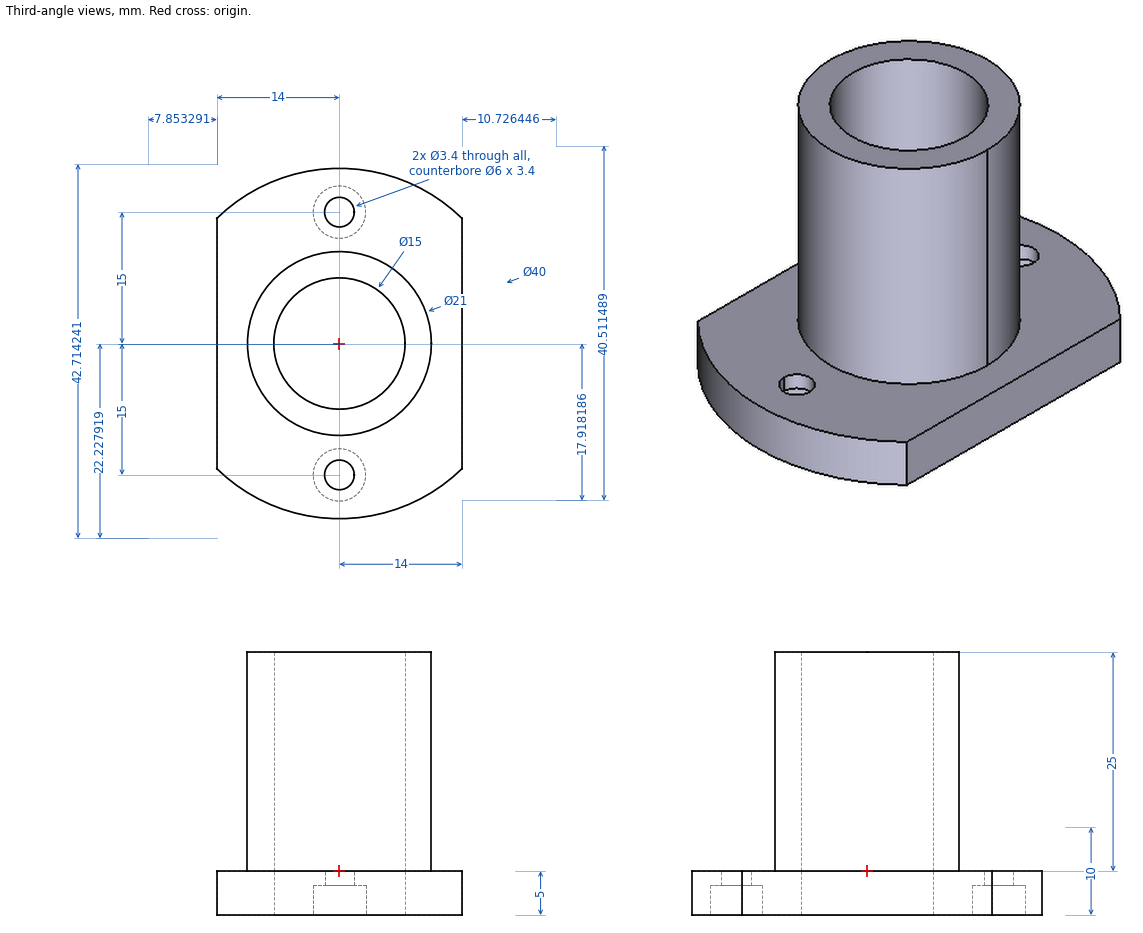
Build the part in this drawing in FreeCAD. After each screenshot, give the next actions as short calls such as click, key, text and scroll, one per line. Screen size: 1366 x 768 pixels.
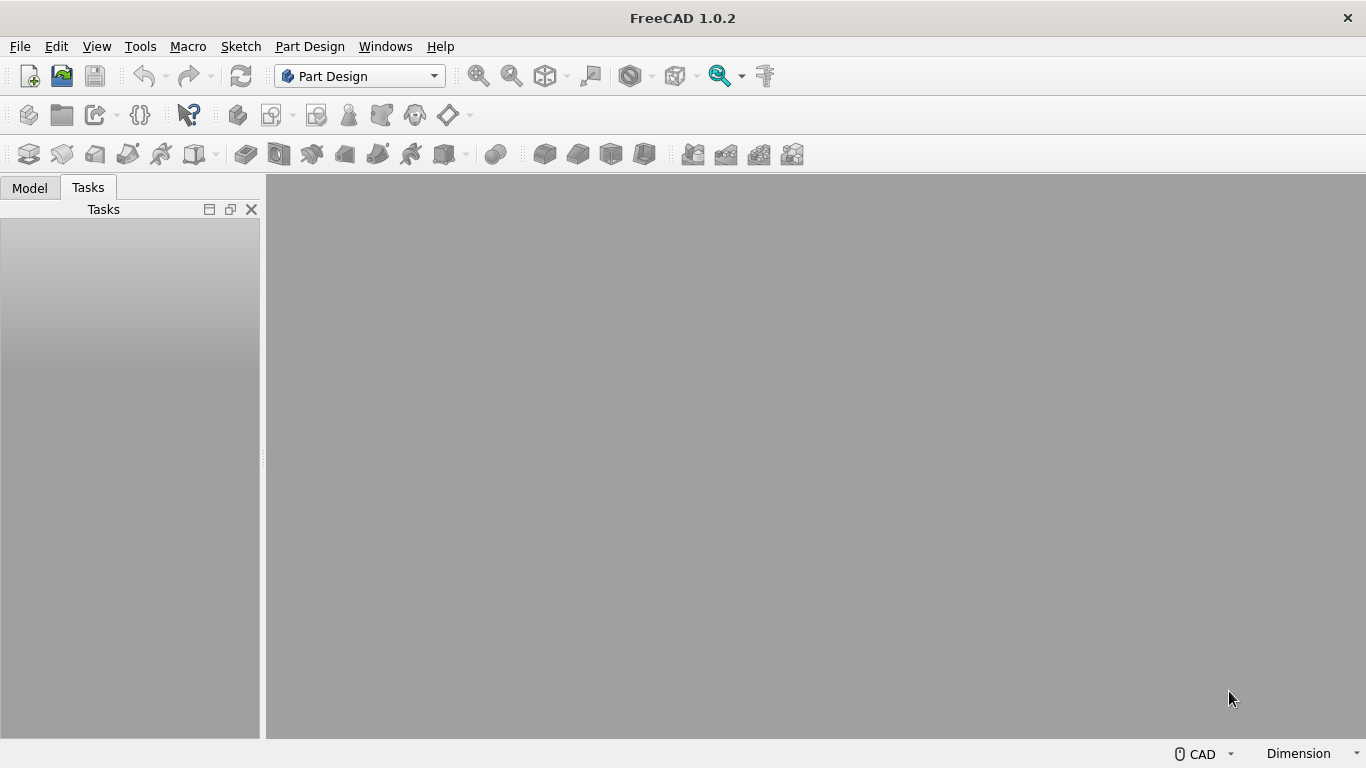
click(29, 76)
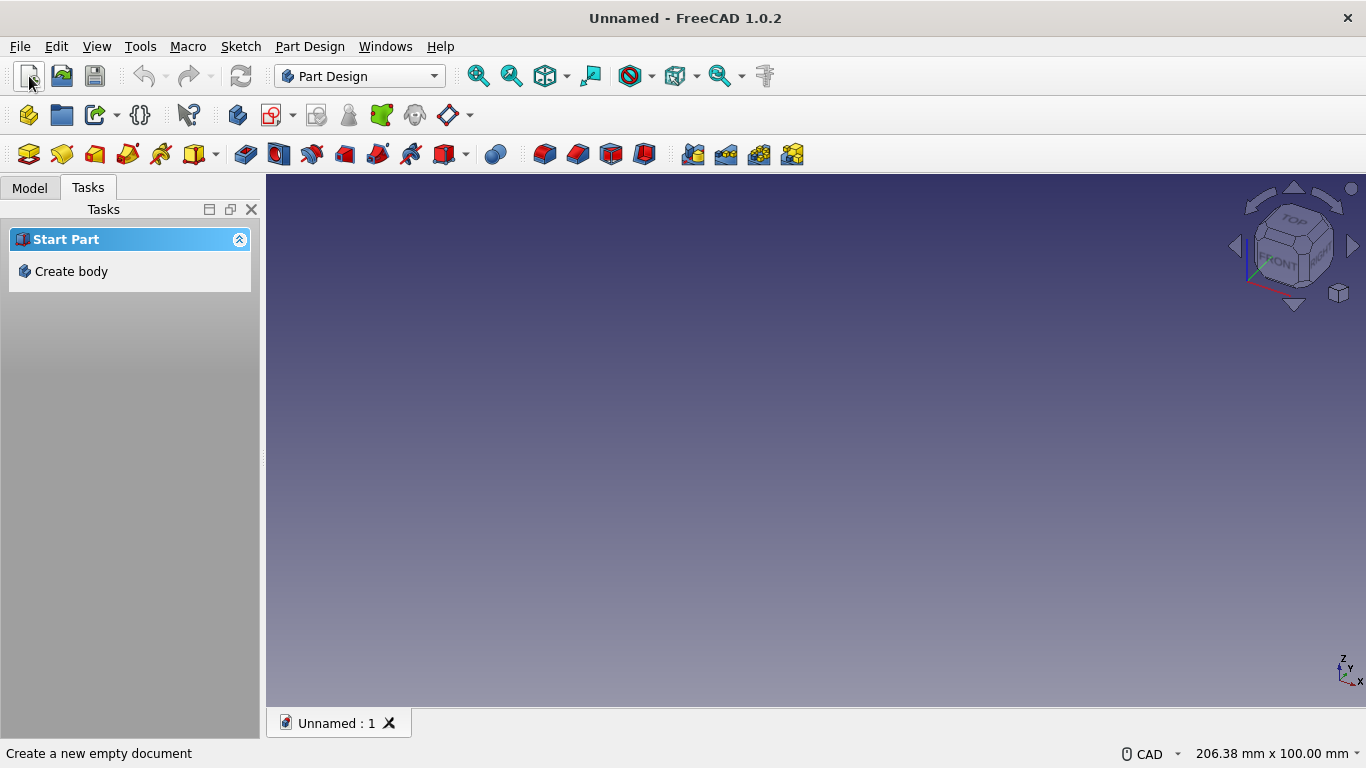
click(270, 116)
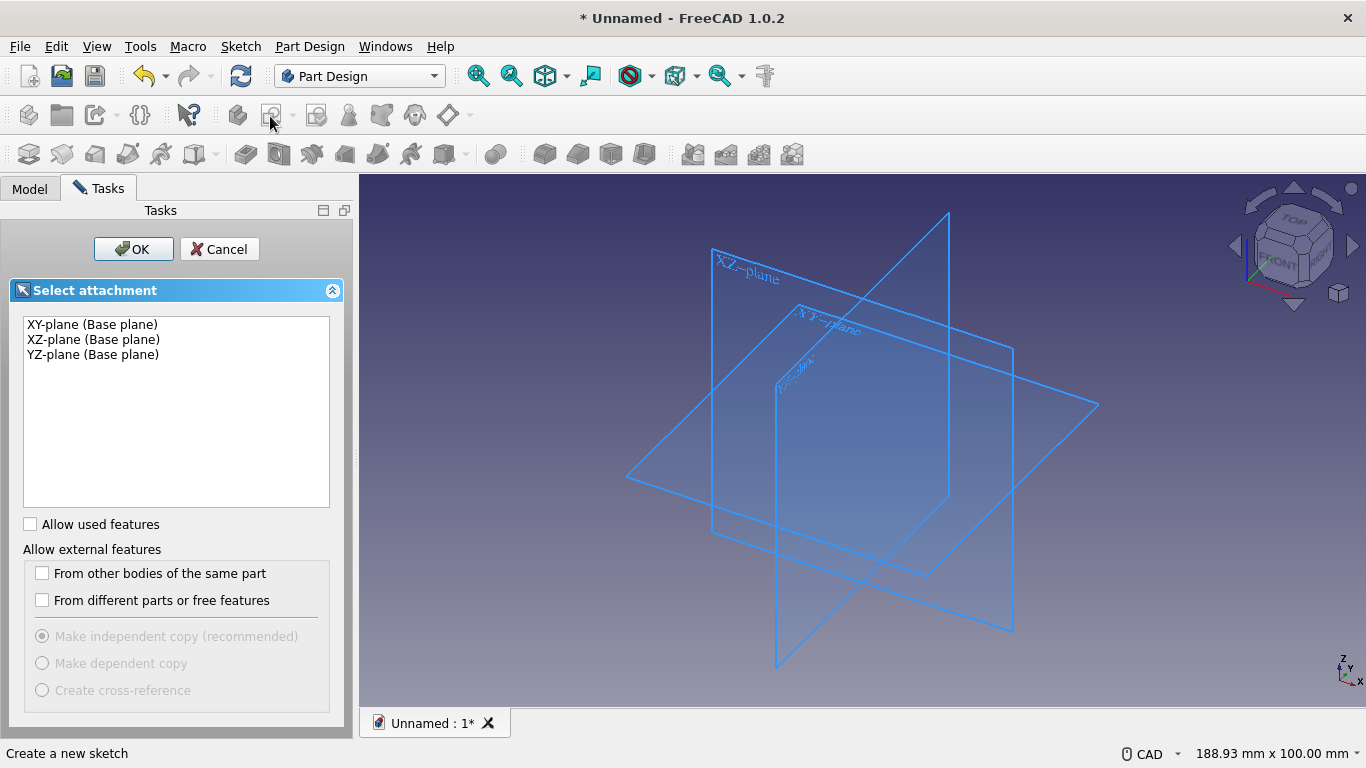
click(84, 324)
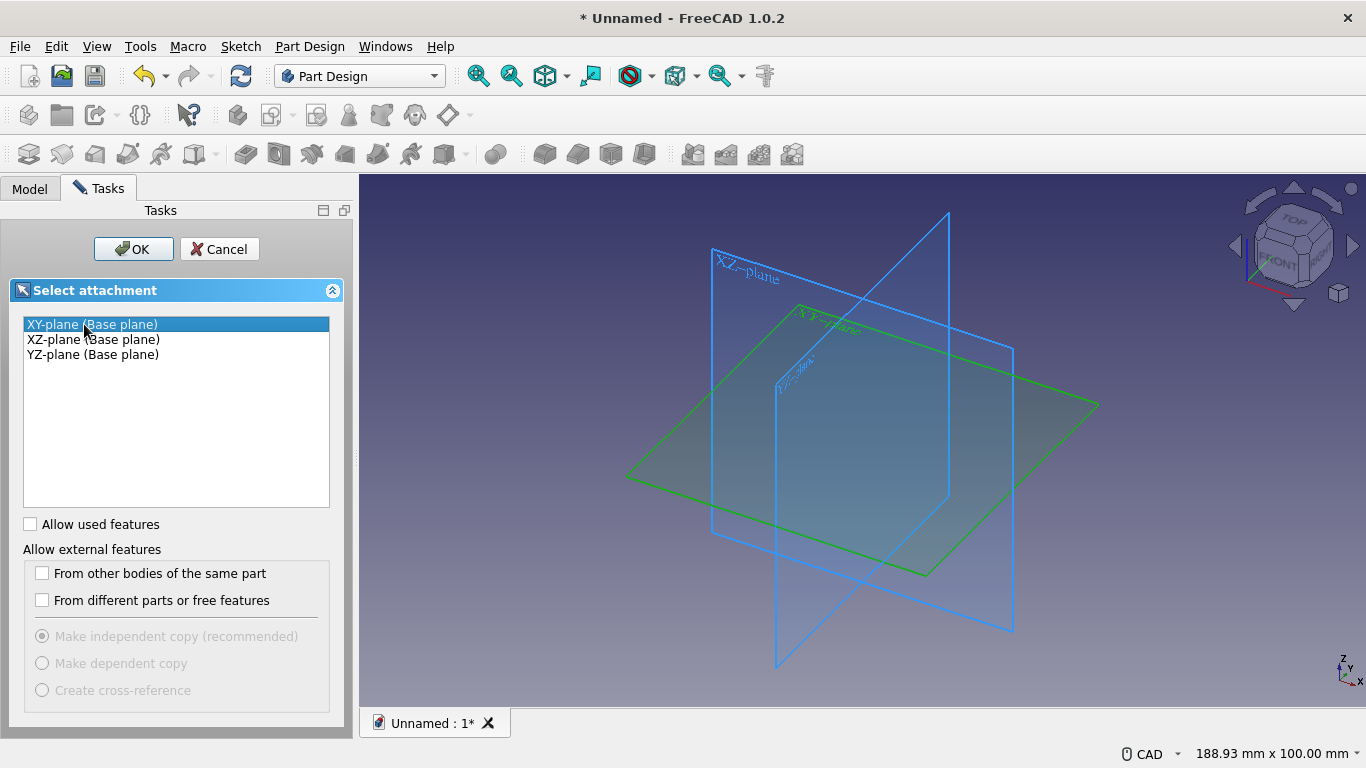
click(134, 249)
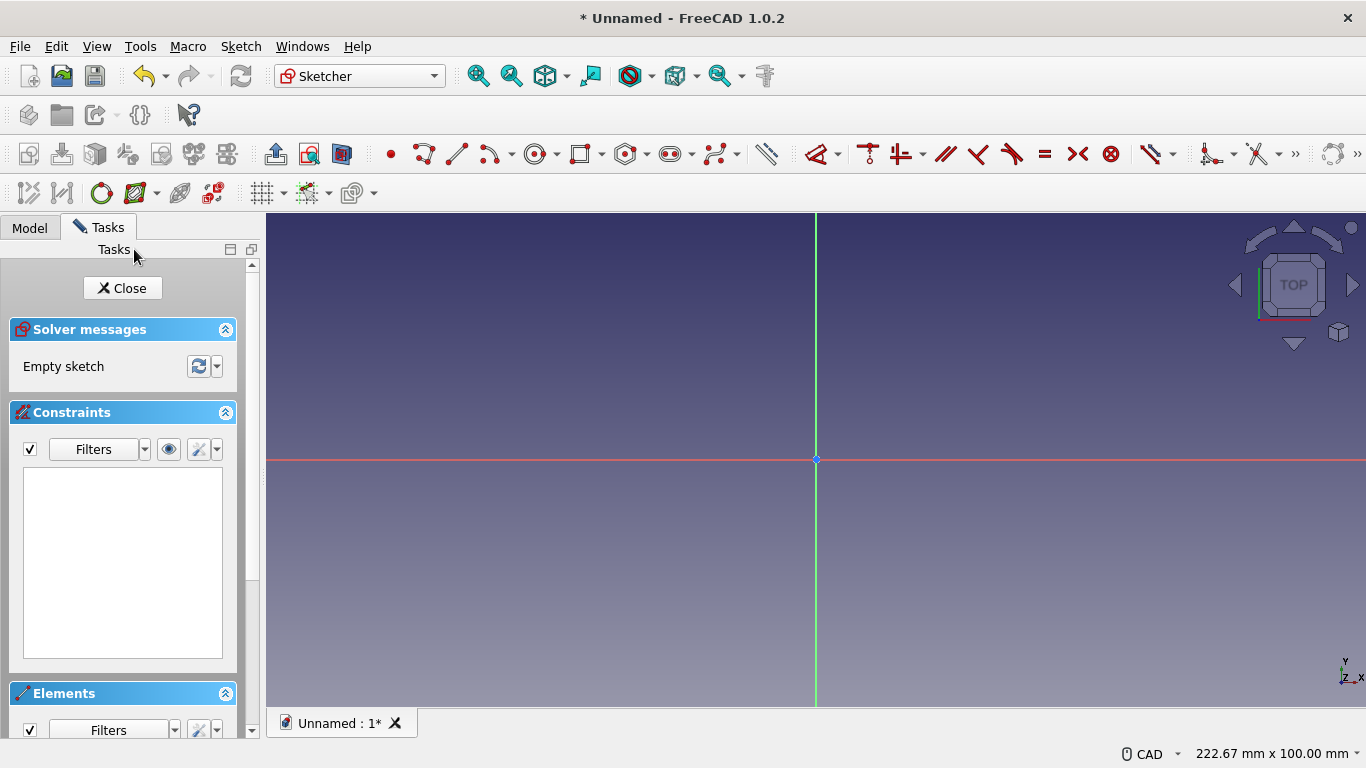
scroll(856, 460, up, 5)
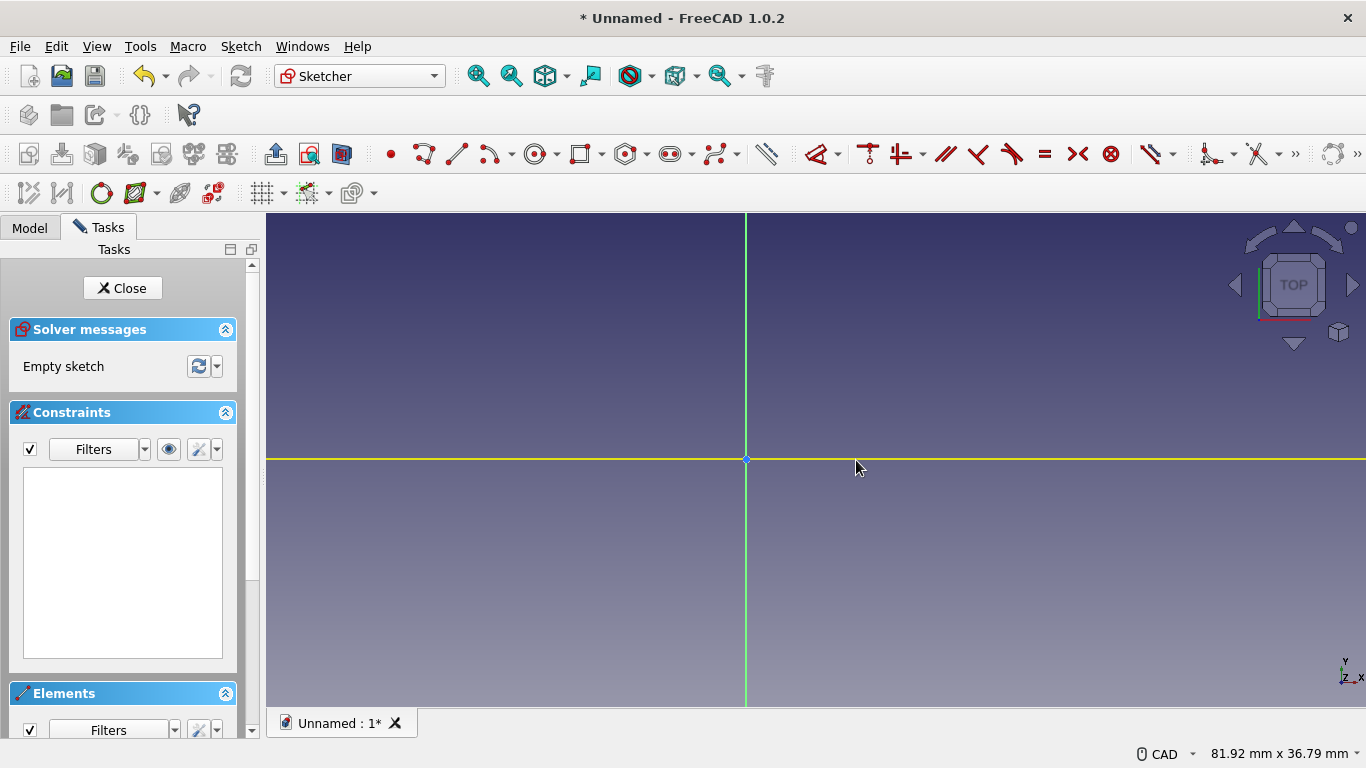
click(534, 154)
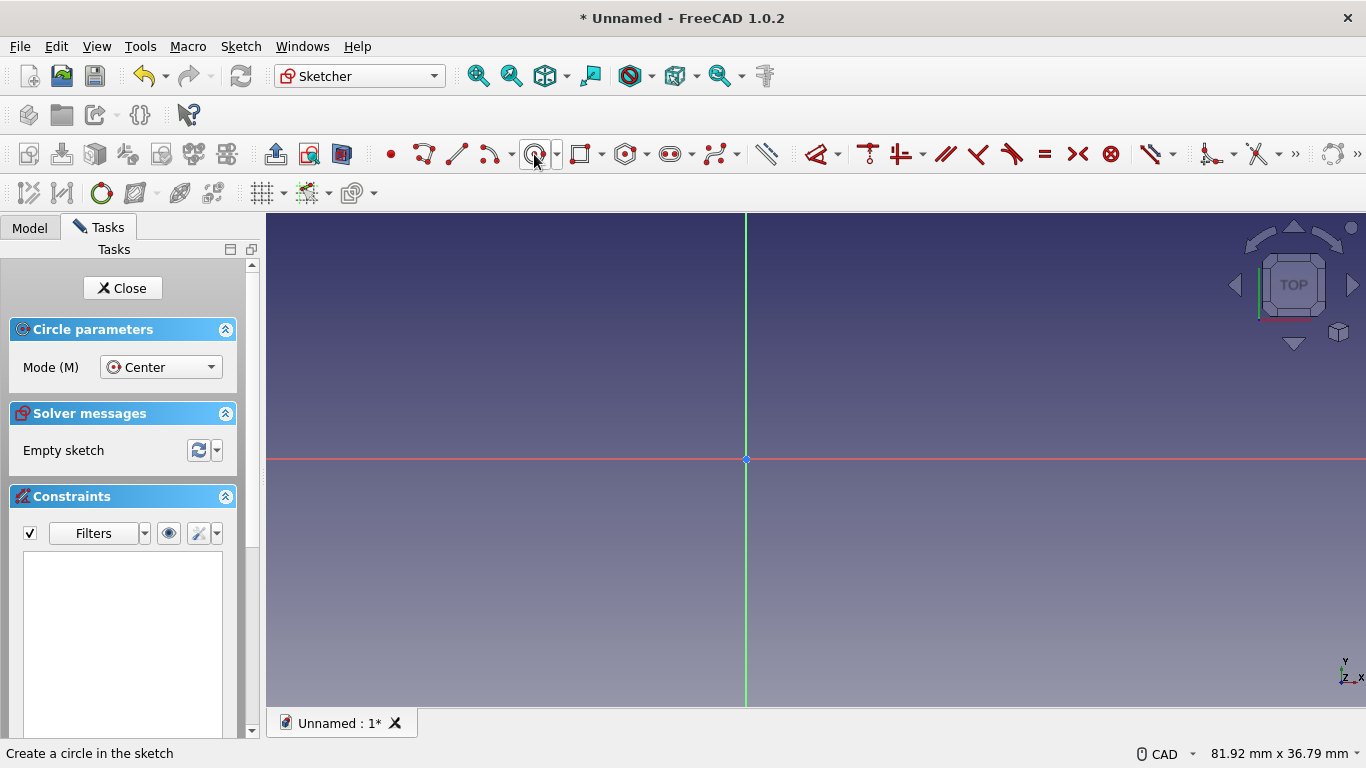
click(746, 459)
move(846, 359)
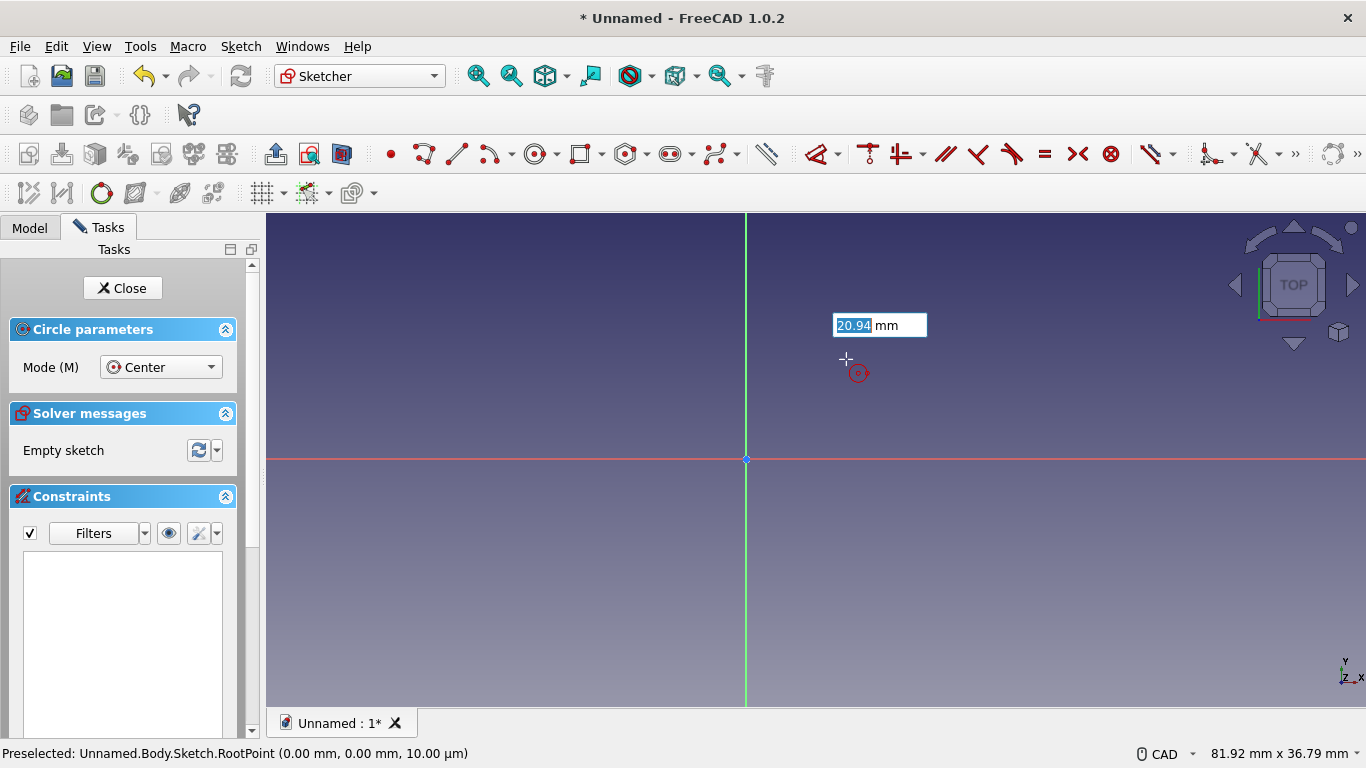
text(21)
key(Return)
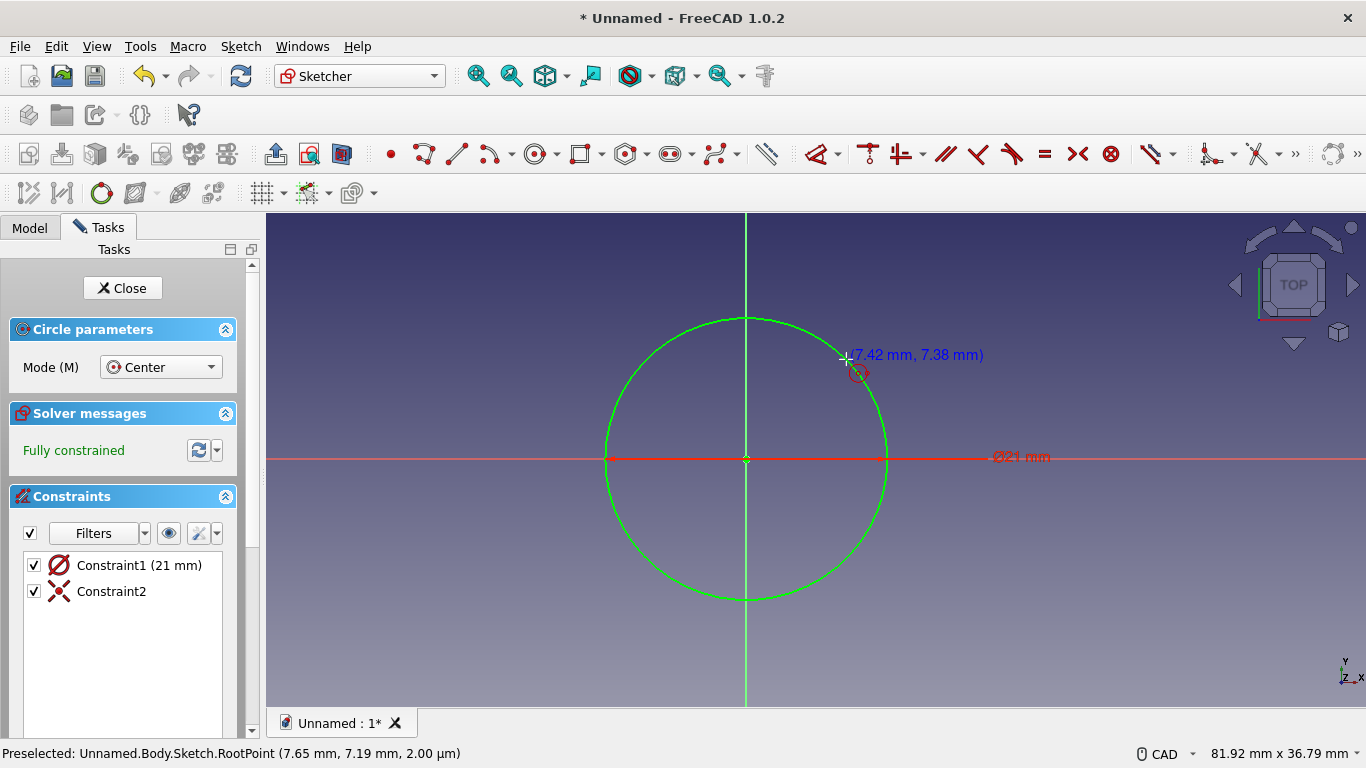
click(746, 459)
move(818, 388)